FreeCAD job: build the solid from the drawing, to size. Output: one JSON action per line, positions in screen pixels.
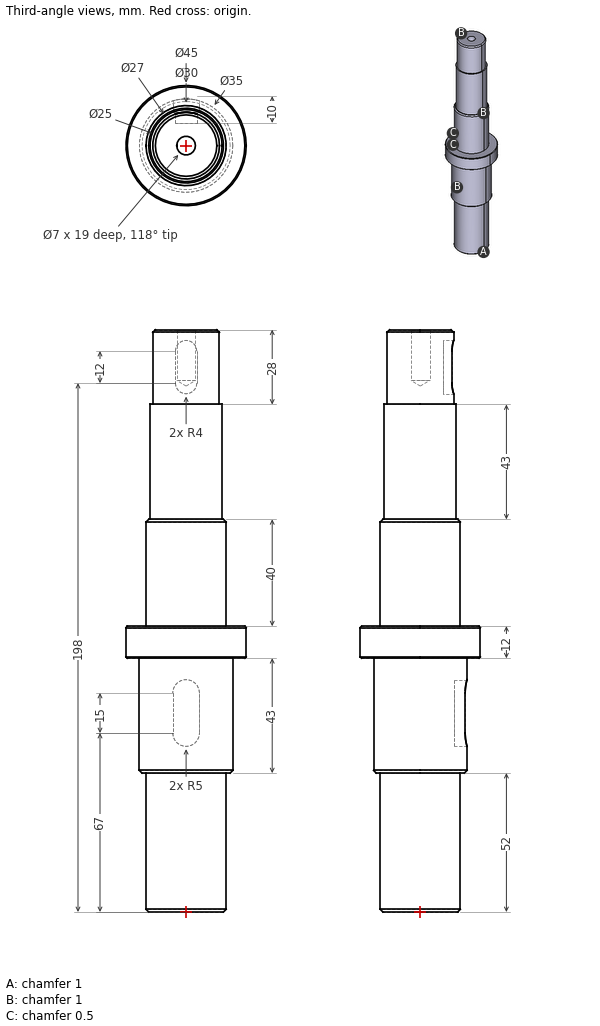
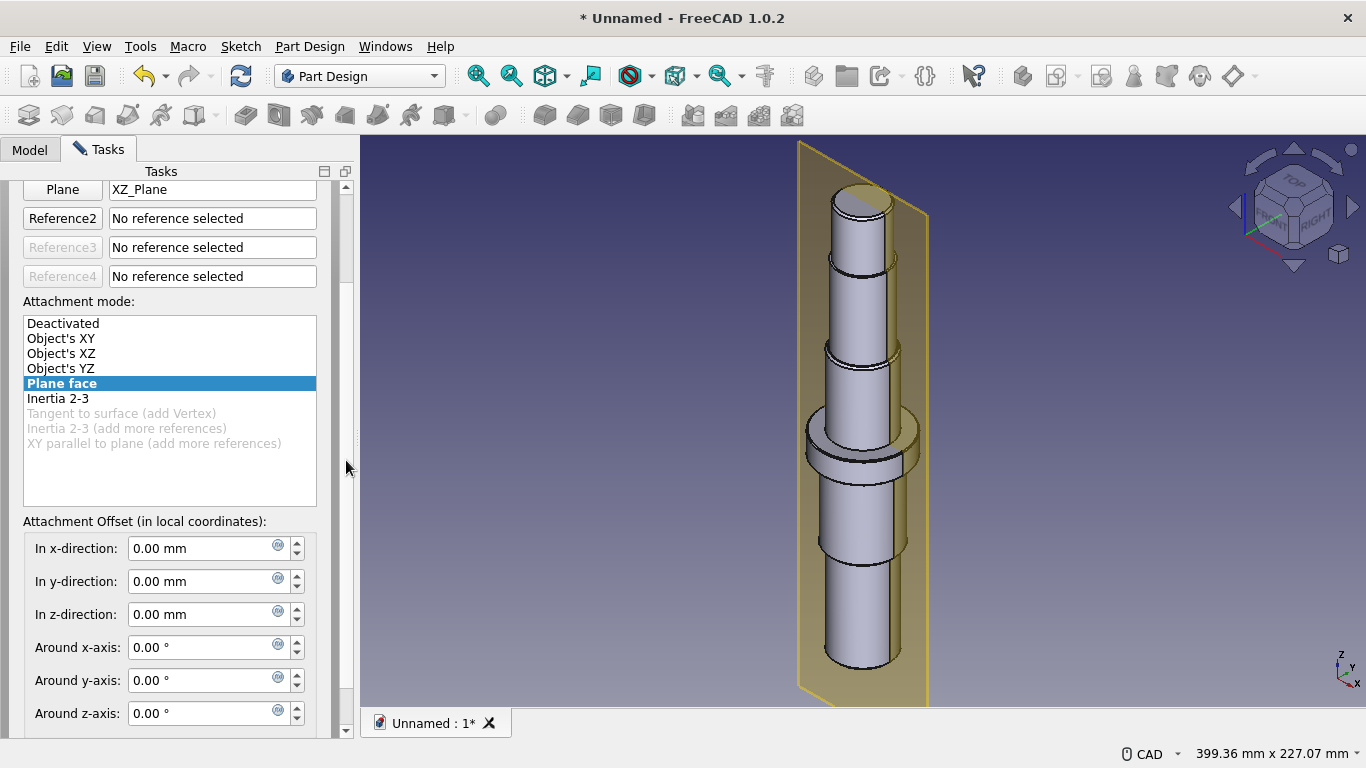
{"action": "triple_click", "coordinate": [210, 614]}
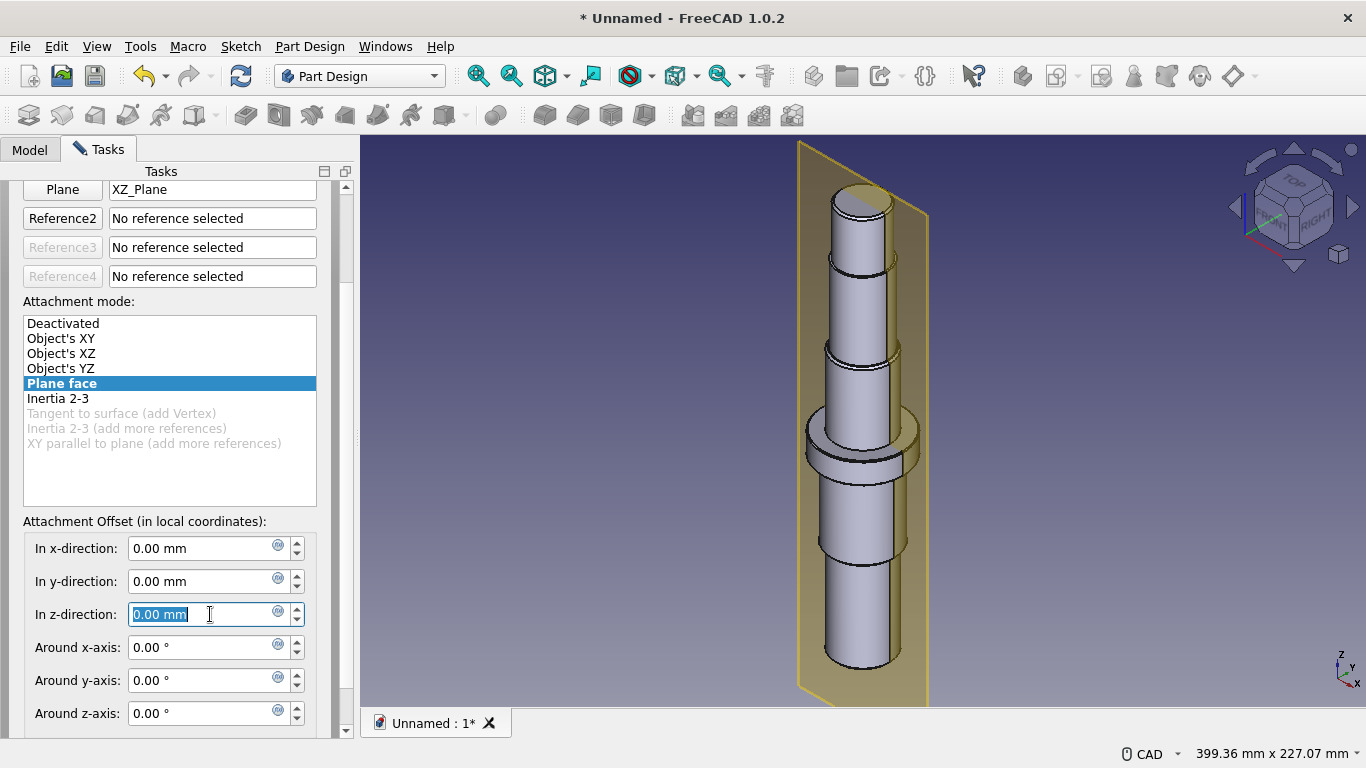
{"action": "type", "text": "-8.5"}
{"action": "key", "text": "Tab"}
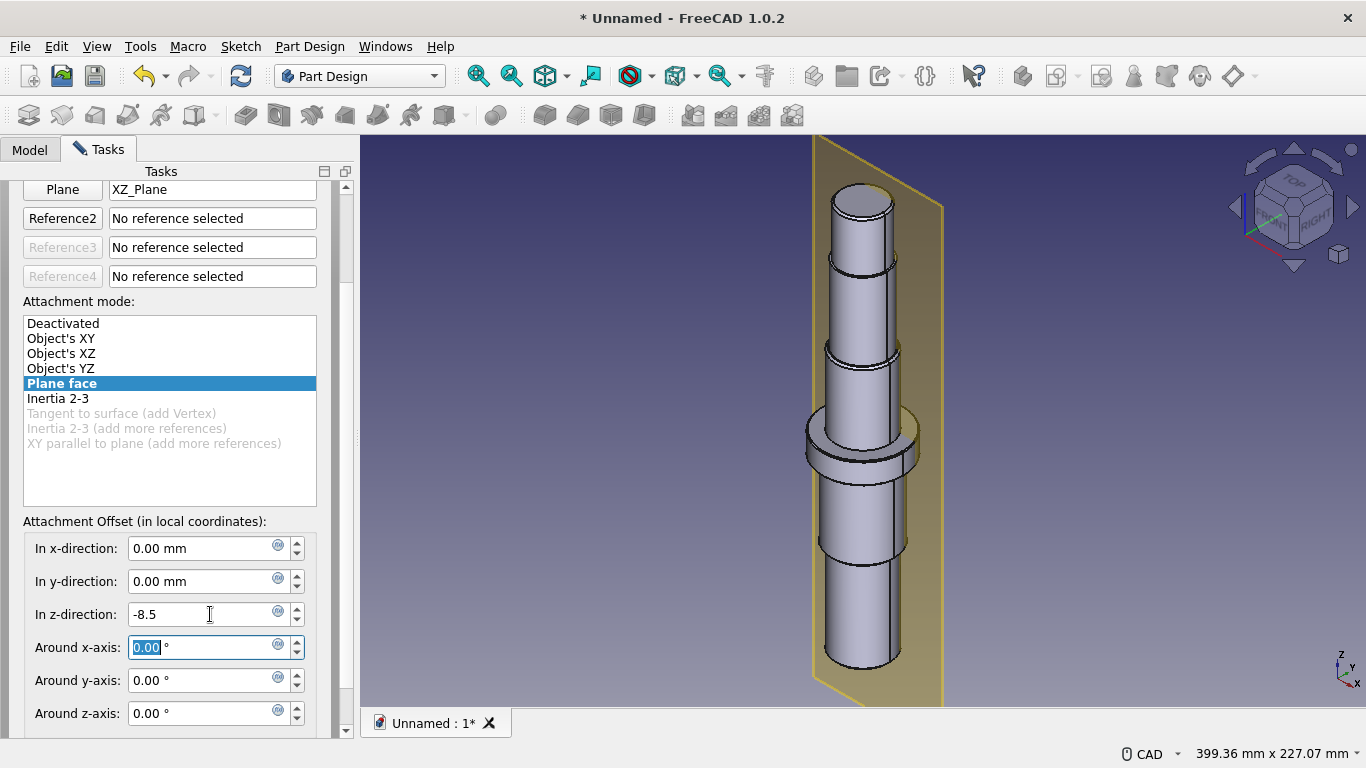
{"action": "scroll", "coordinate": [346, 460], "scroll_direction": "up", "scroll_amount": 3}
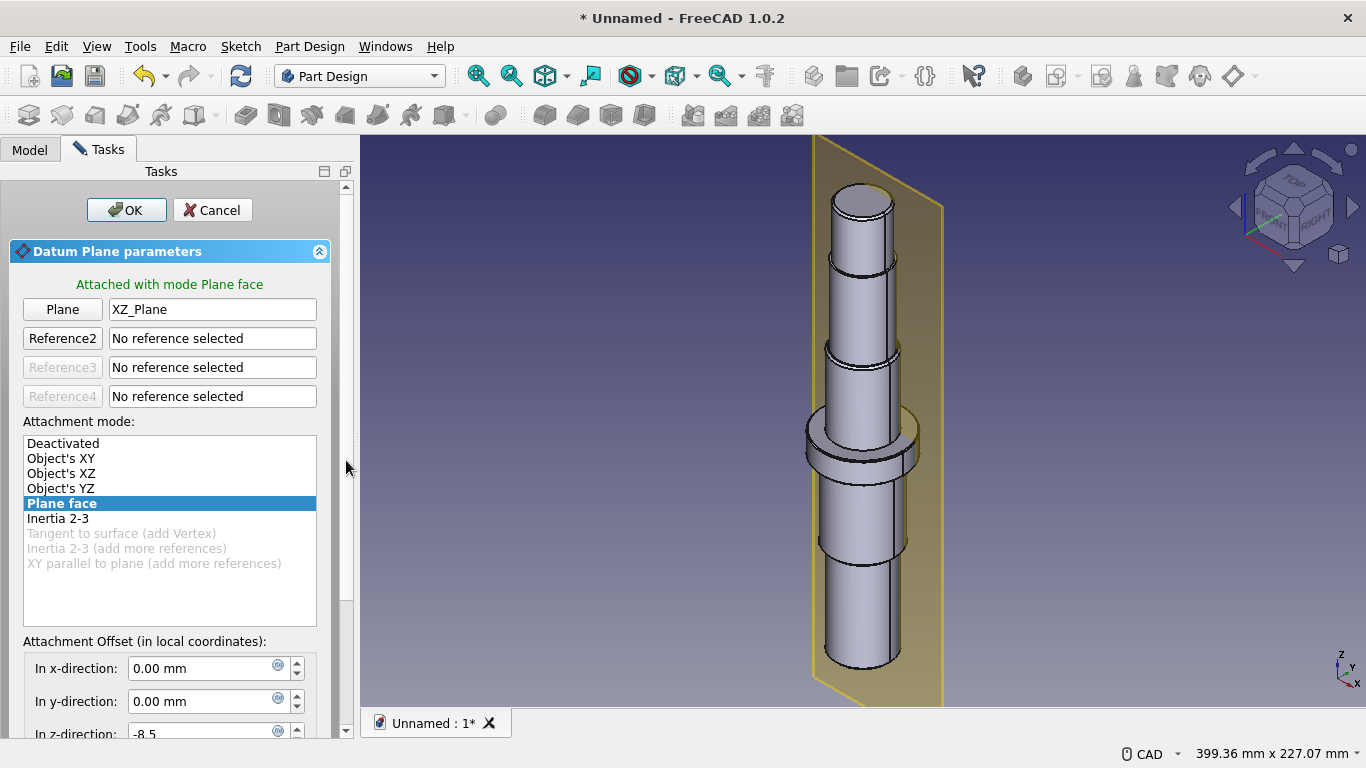
{"action": "left_click", "coordinate": [127, 210]}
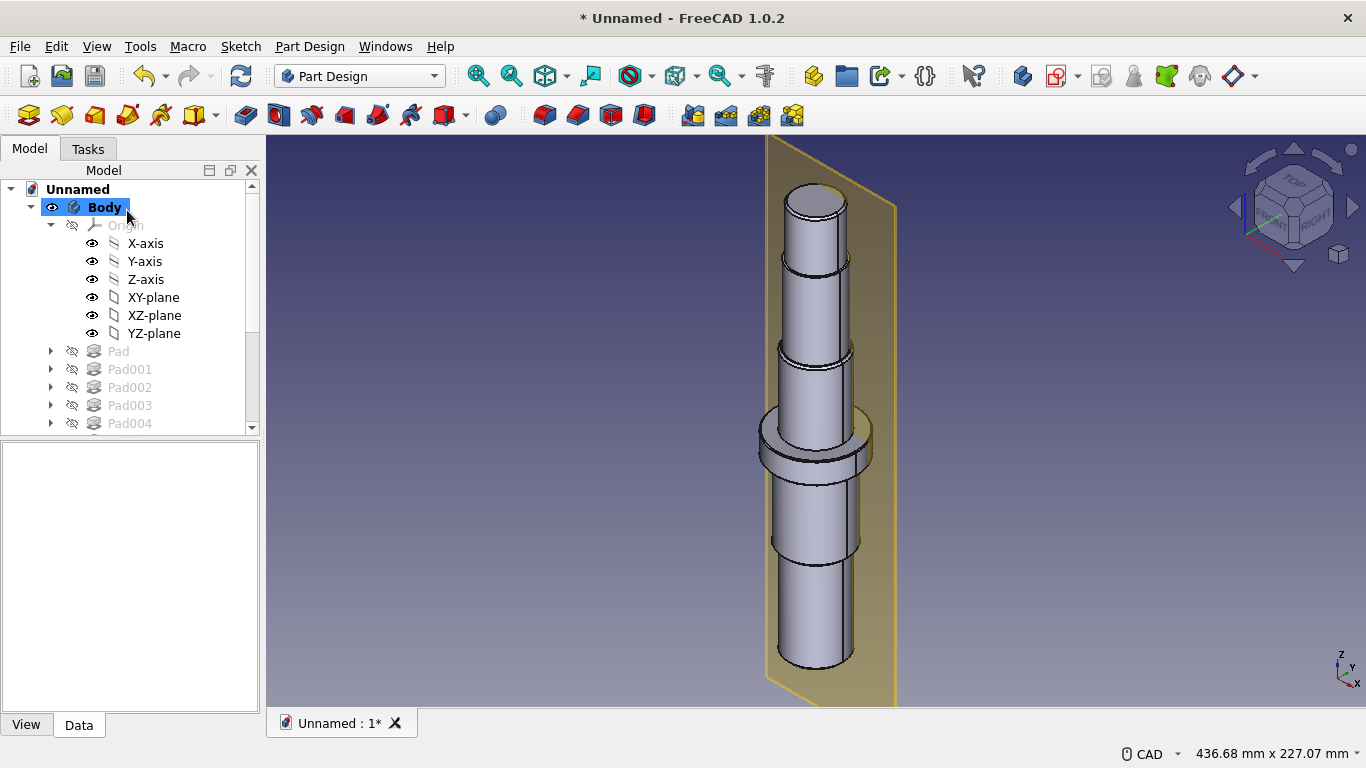
{"action": "scroll", "coordinate": [101, 311], "scroll_direction": "down", "scroll_amount": 3}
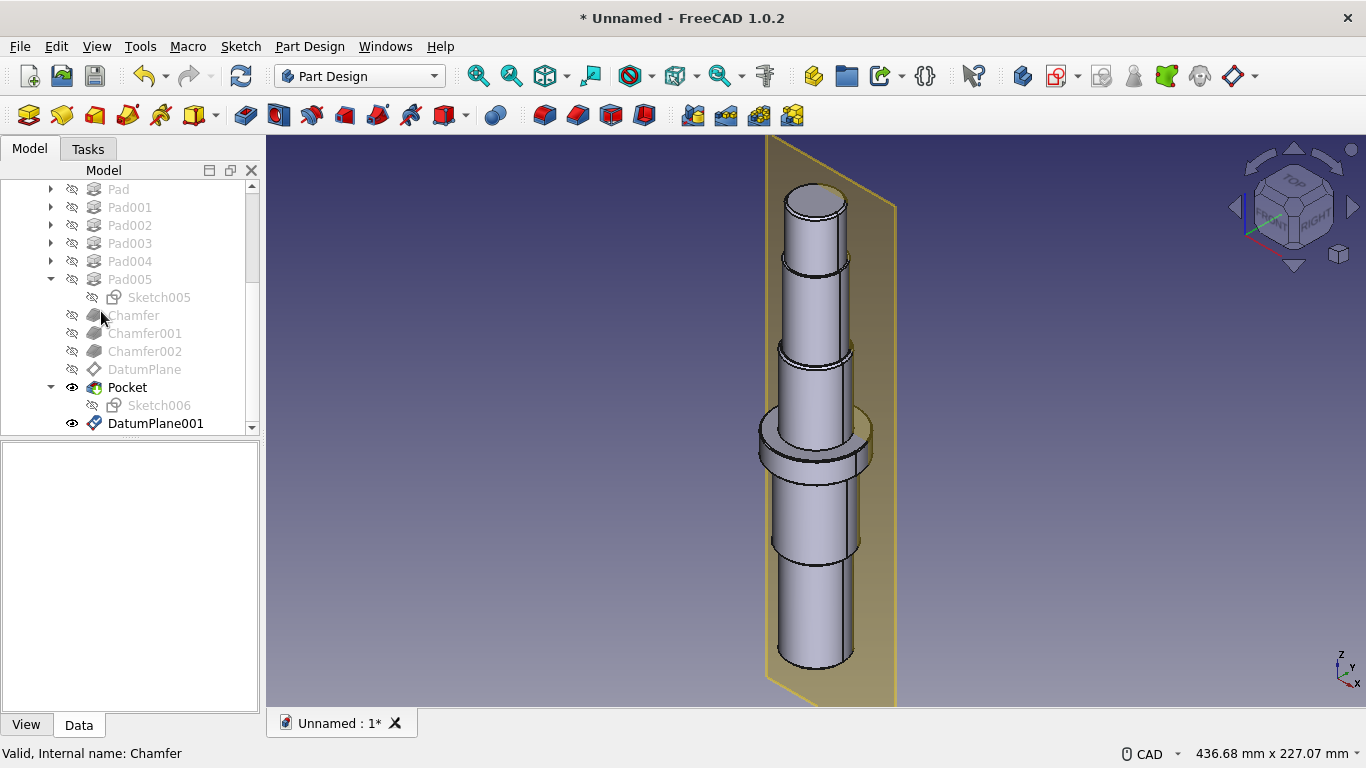
{"action": "left_click", "coordinate": [117, 423]}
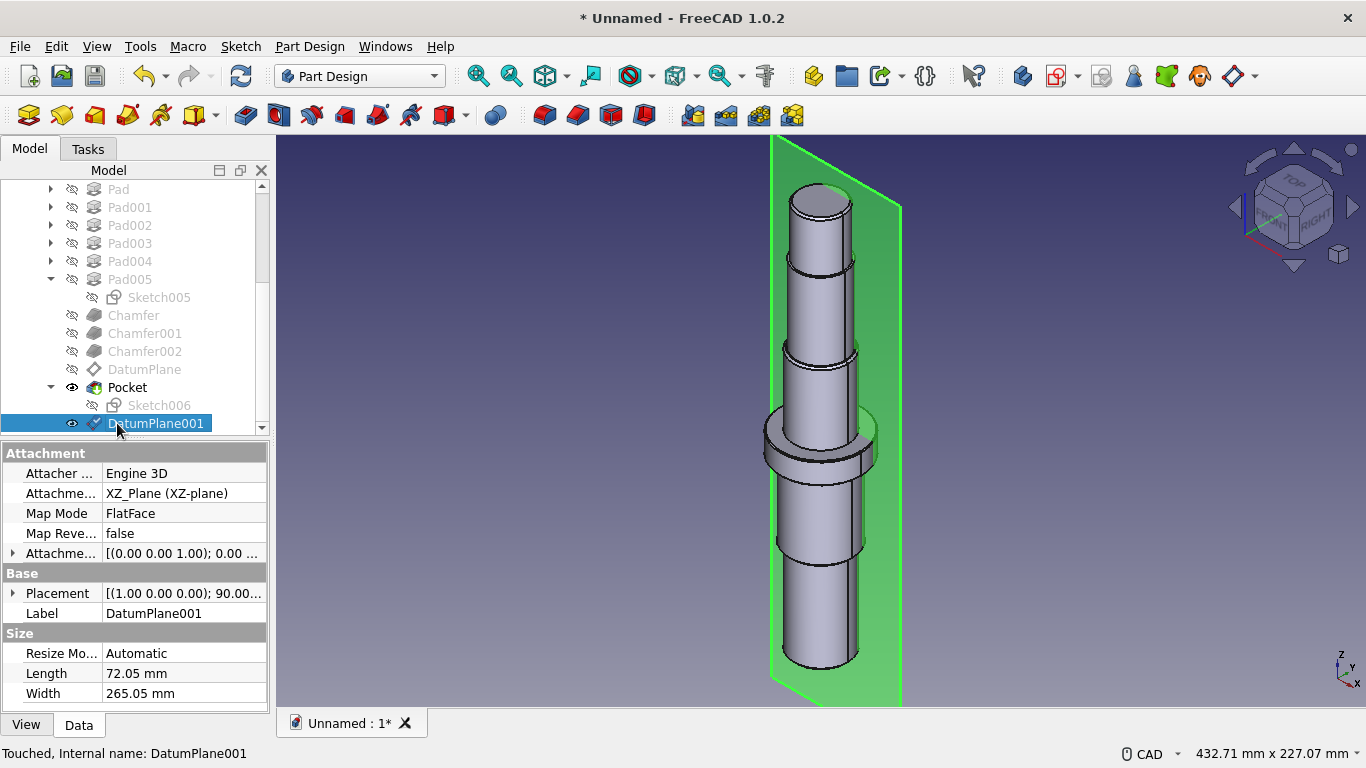
{"action": "left_click", "coordinate": [1056, 76]}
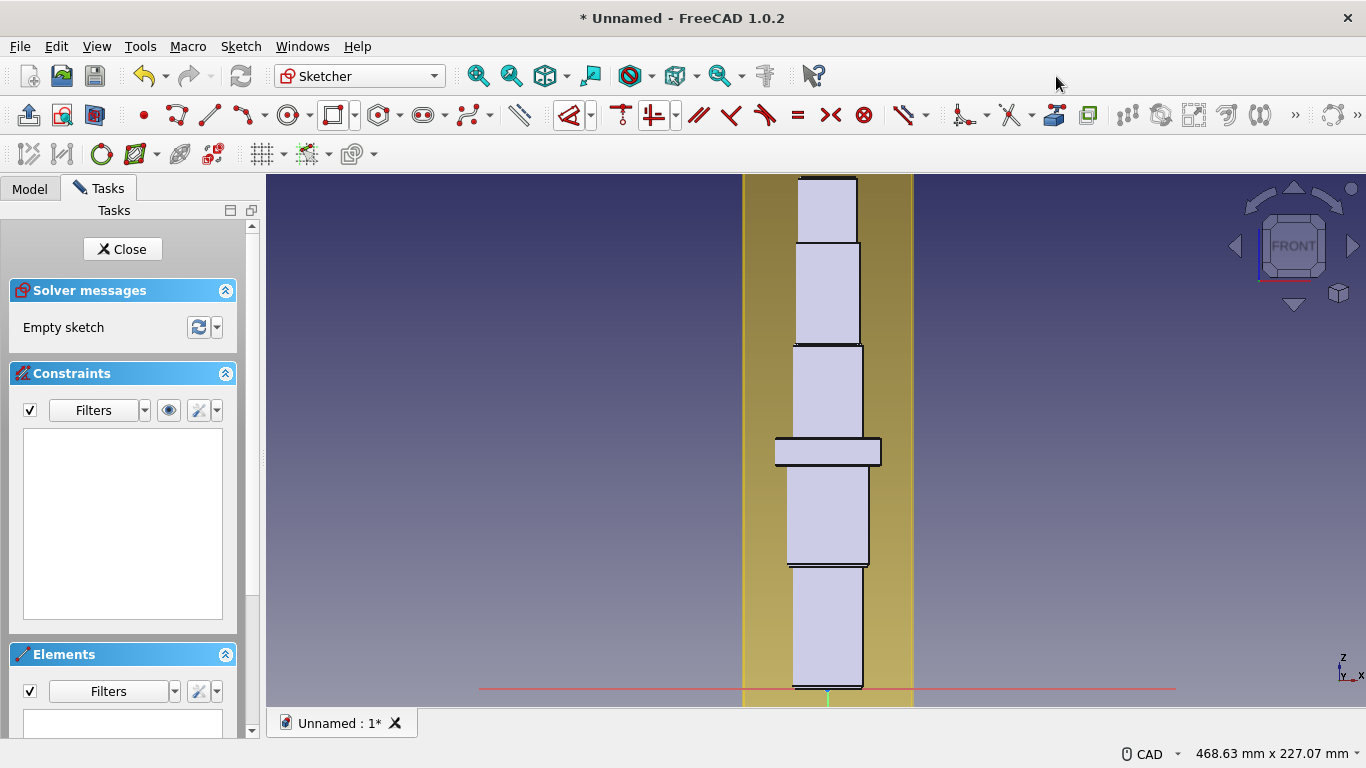
{"action": "left_click", "coordinate": [95, 116]}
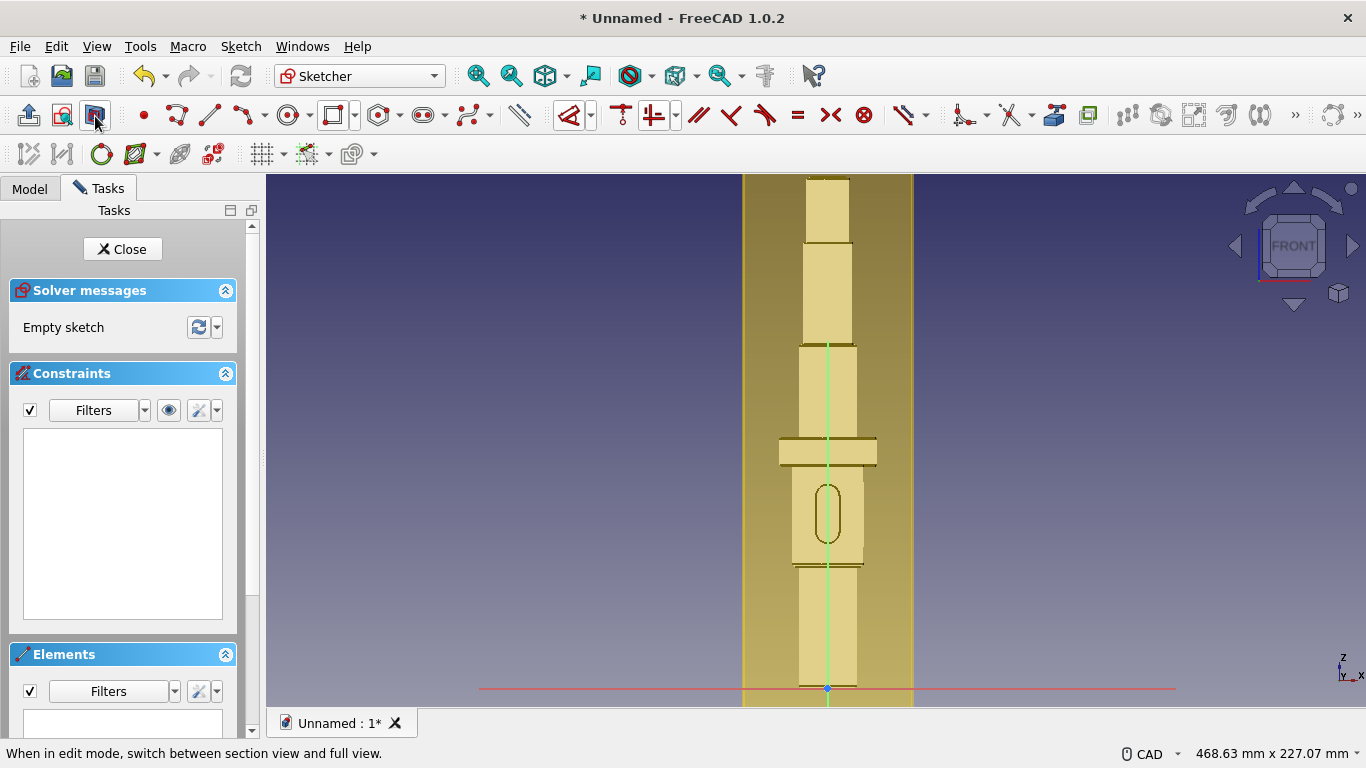
{"action": "scroll", "coordinate": [748, 440], "scroll_direction": "down", "scroll_amount": 5}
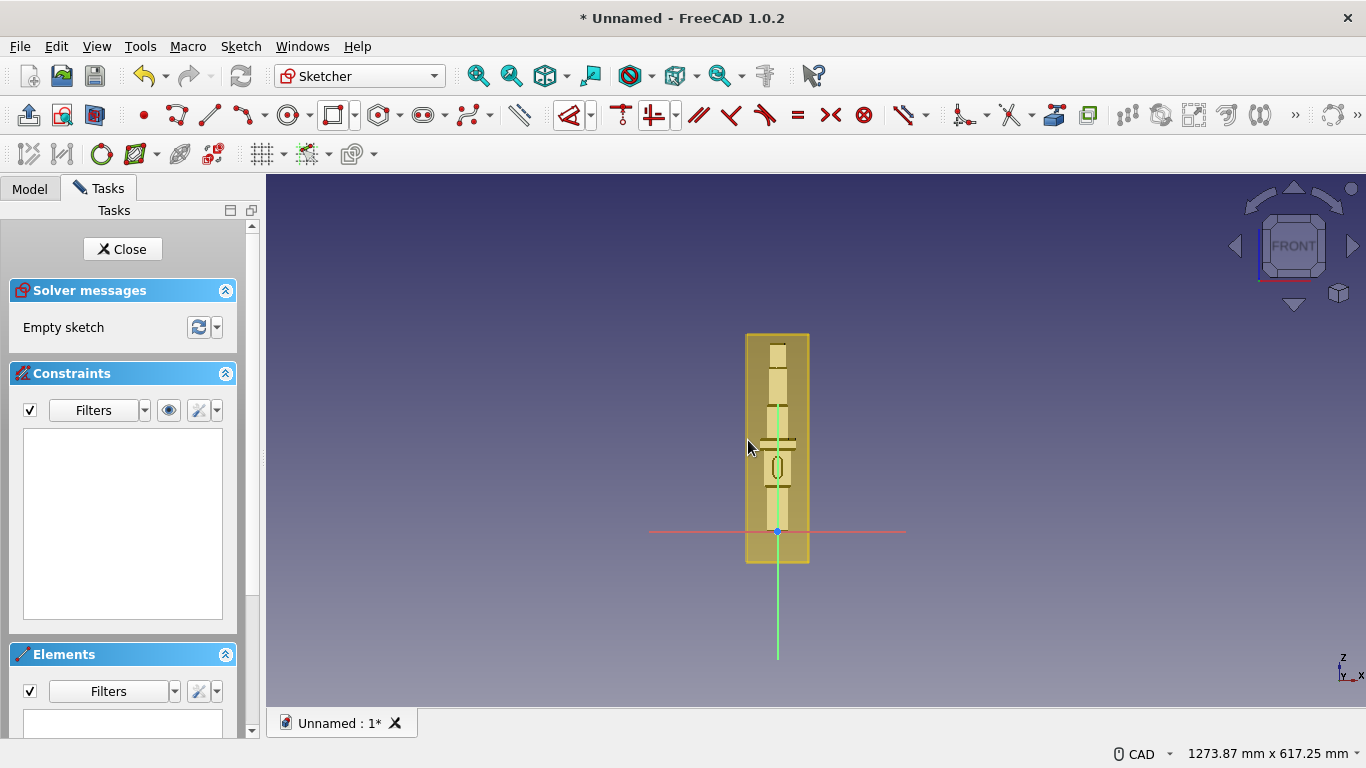
{"action": "scroll", "coordinate": [779, 351], "scroll_direction": "up", "scroll_amount": 15}